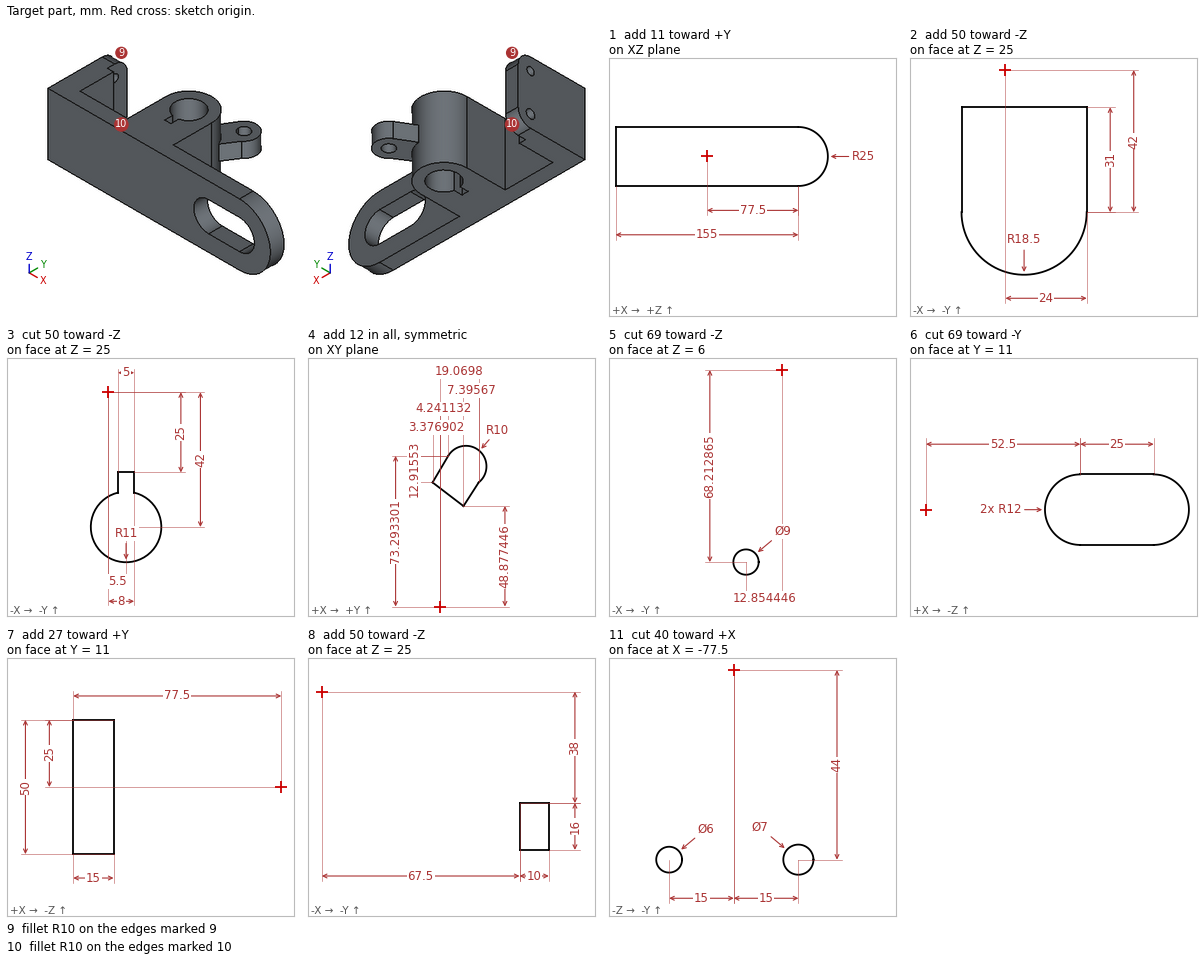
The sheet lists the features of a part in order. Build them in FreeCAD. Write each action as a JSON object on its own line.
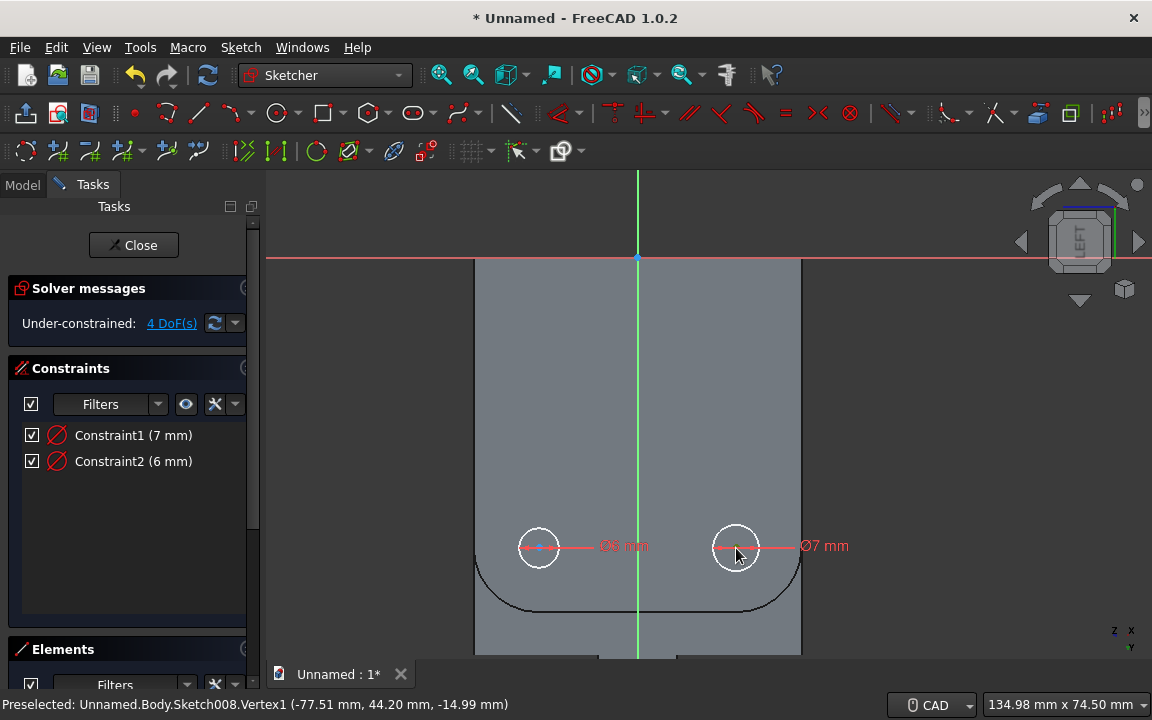
{"action": "left_click", "coordinate": [539, 548]}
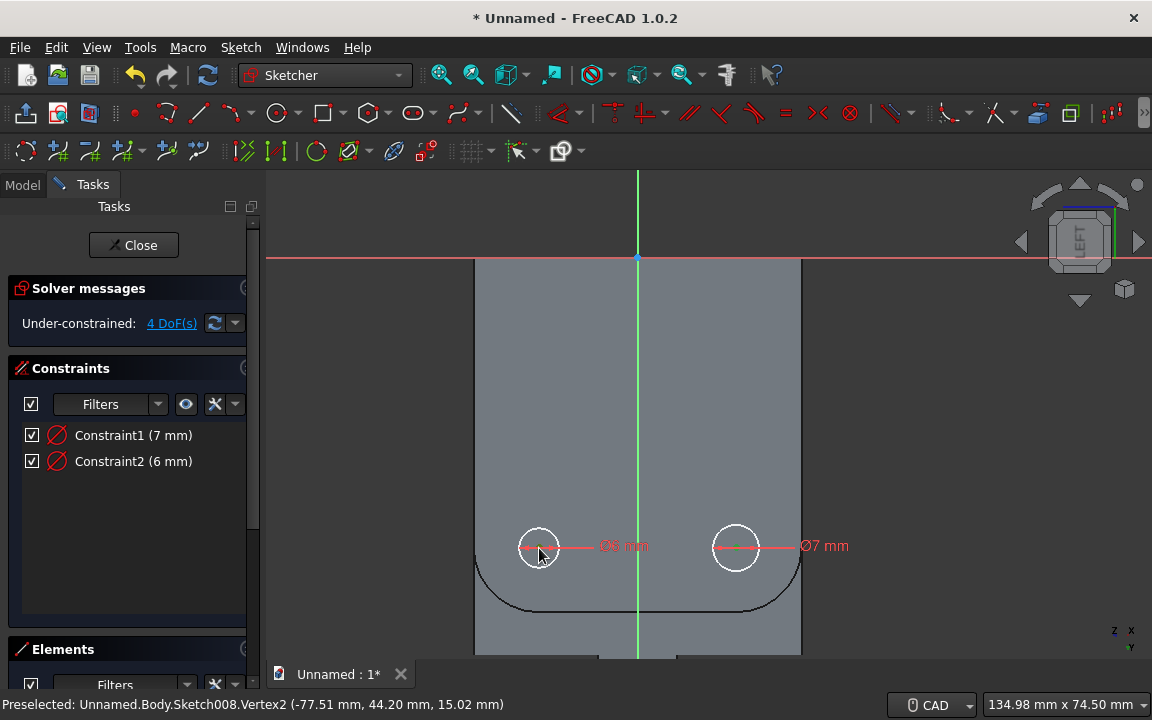
{"action": "left_click", "coordinate": [668, 114]}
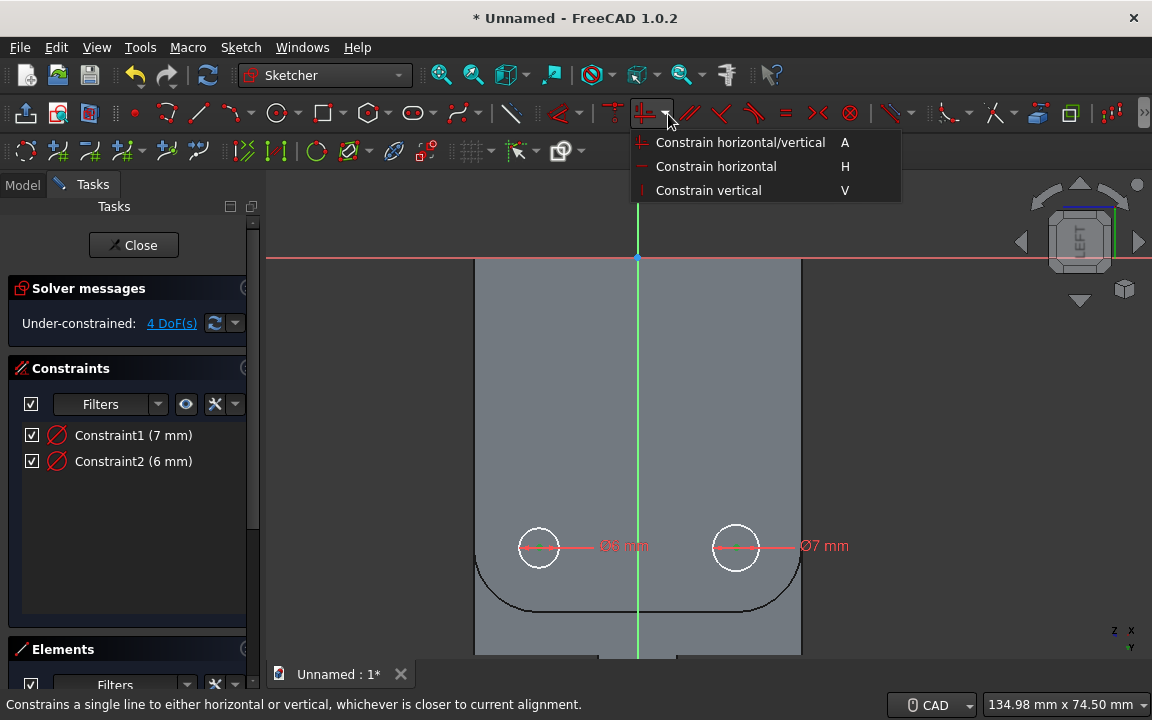
{"action": "left_click", "coordinate": [766, 166]}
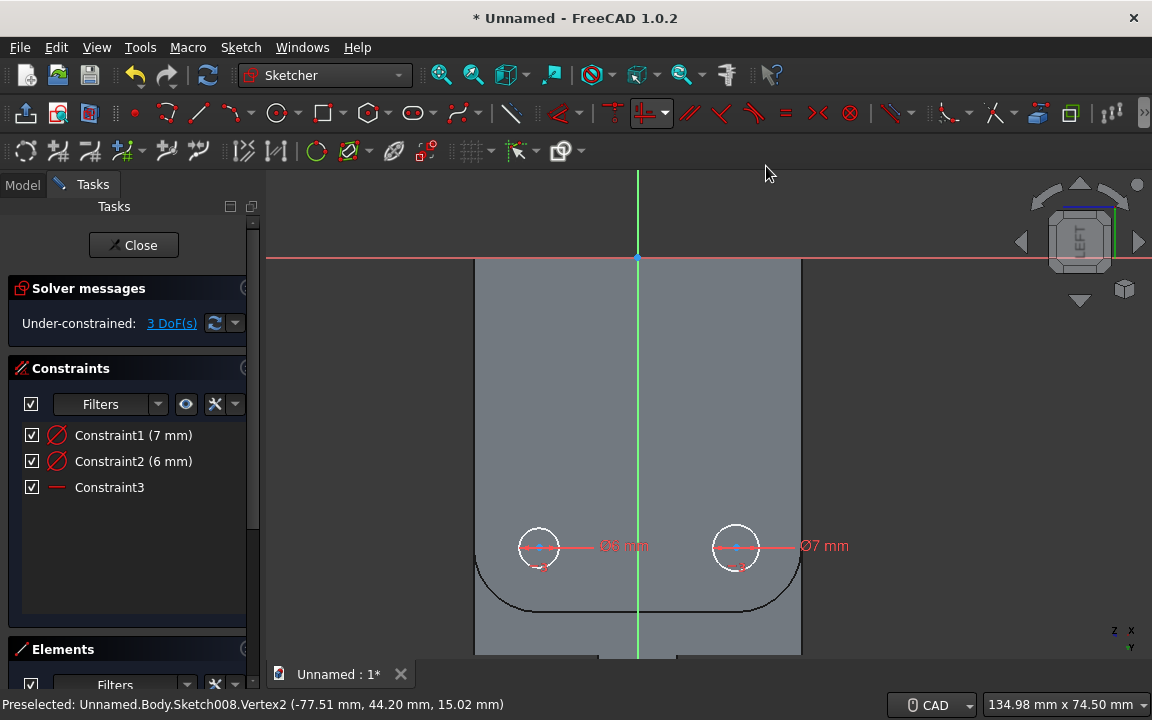
{"action": "left_click", "coordinate": [558, 114]}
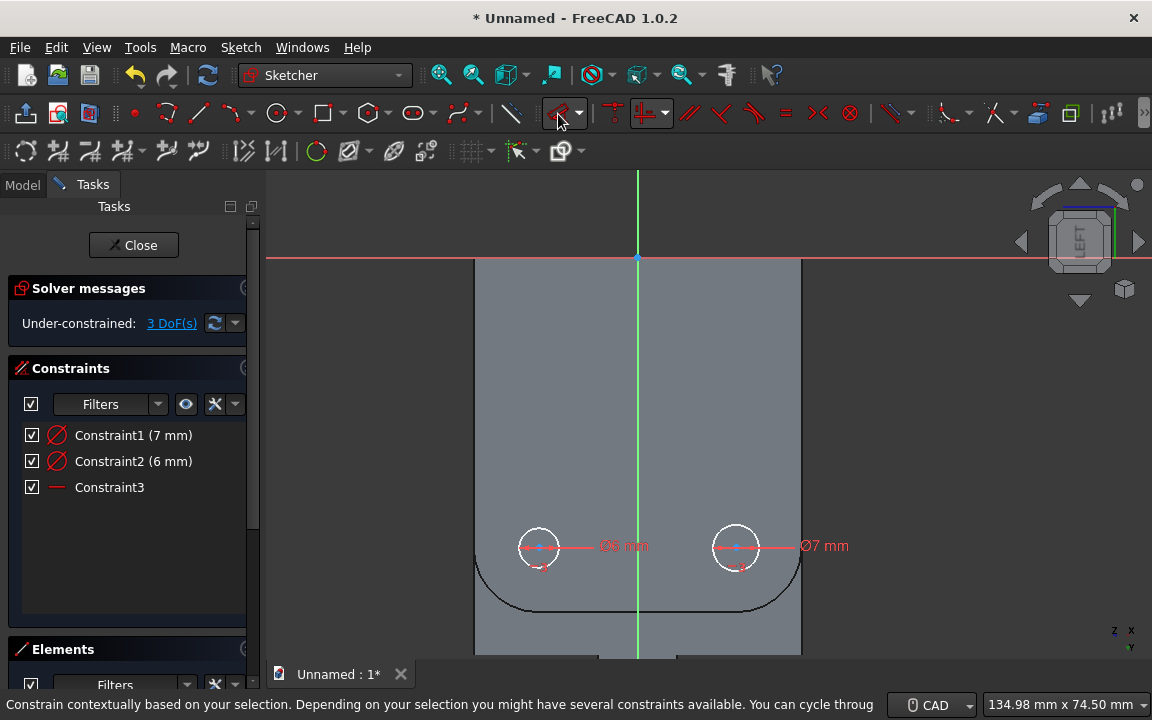
{"action": "left_click", "coordinate": [736, 548]}
{"action": "left_click", "coordinate": [687, 224]}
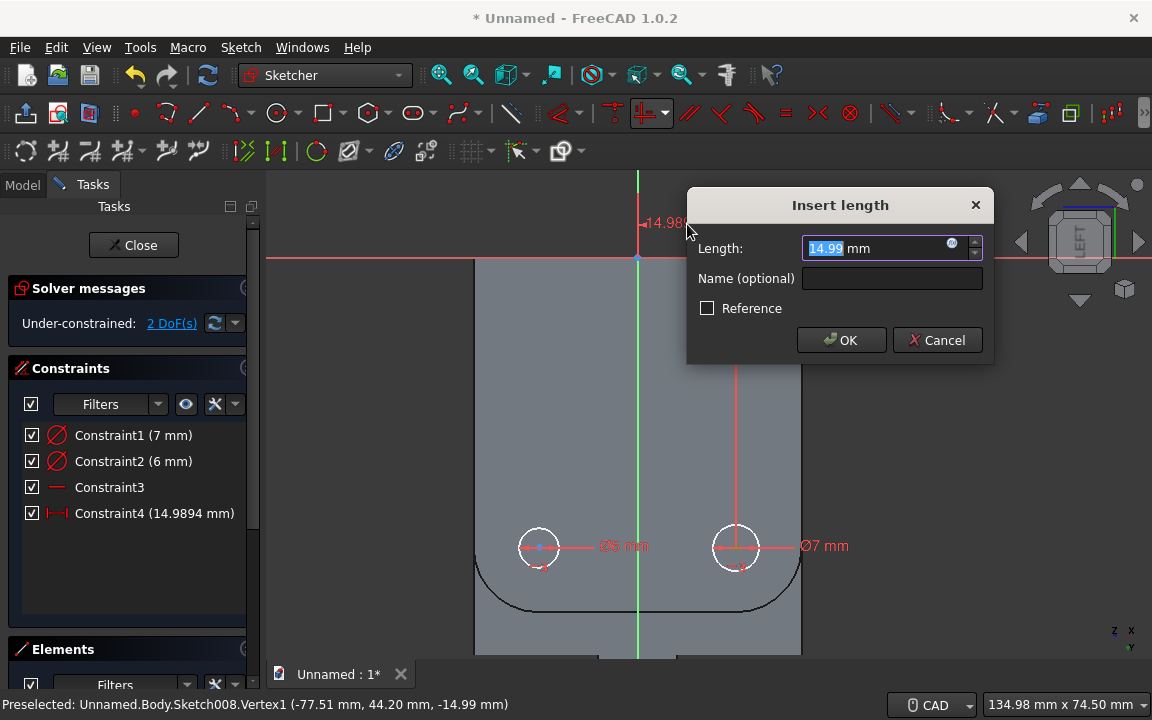
{"action": "type", "text": "15"}
{"action": "key", "text": "Return"}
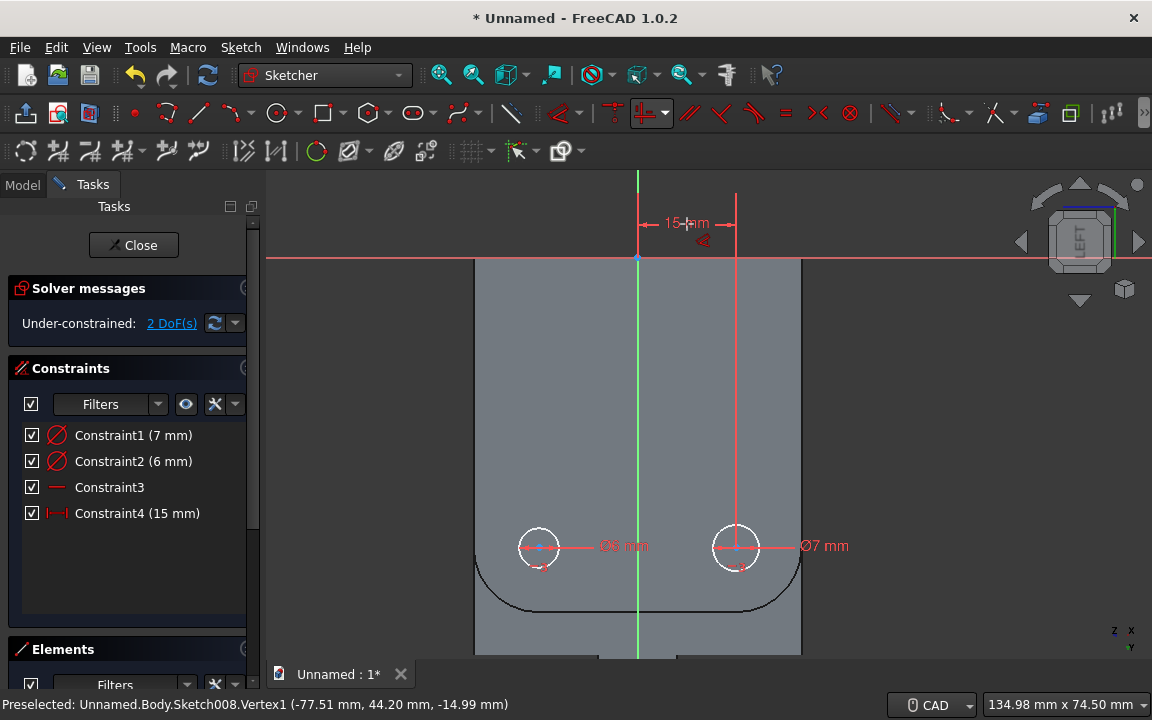
{"action": "left_click", "coordinate": [736, 548]}
{"action": "left_click", "coordinate": [770, 403]}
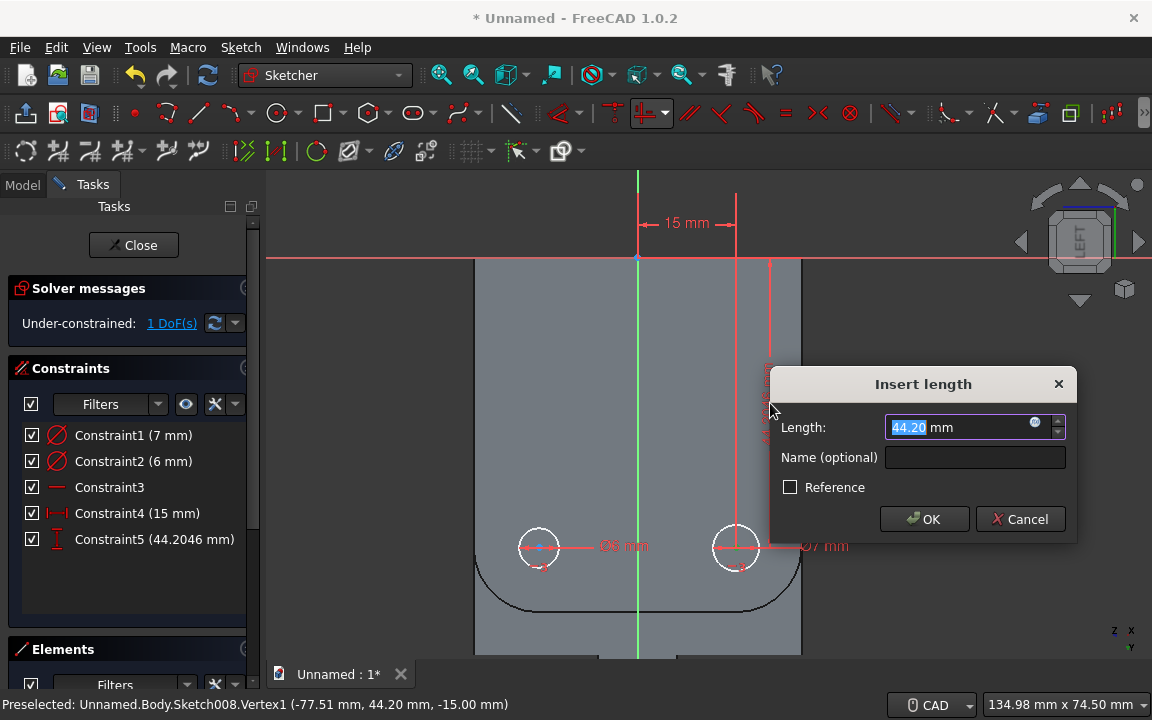
{"action": "type", "text": "44"}
{"action": "key", "text": "Return"}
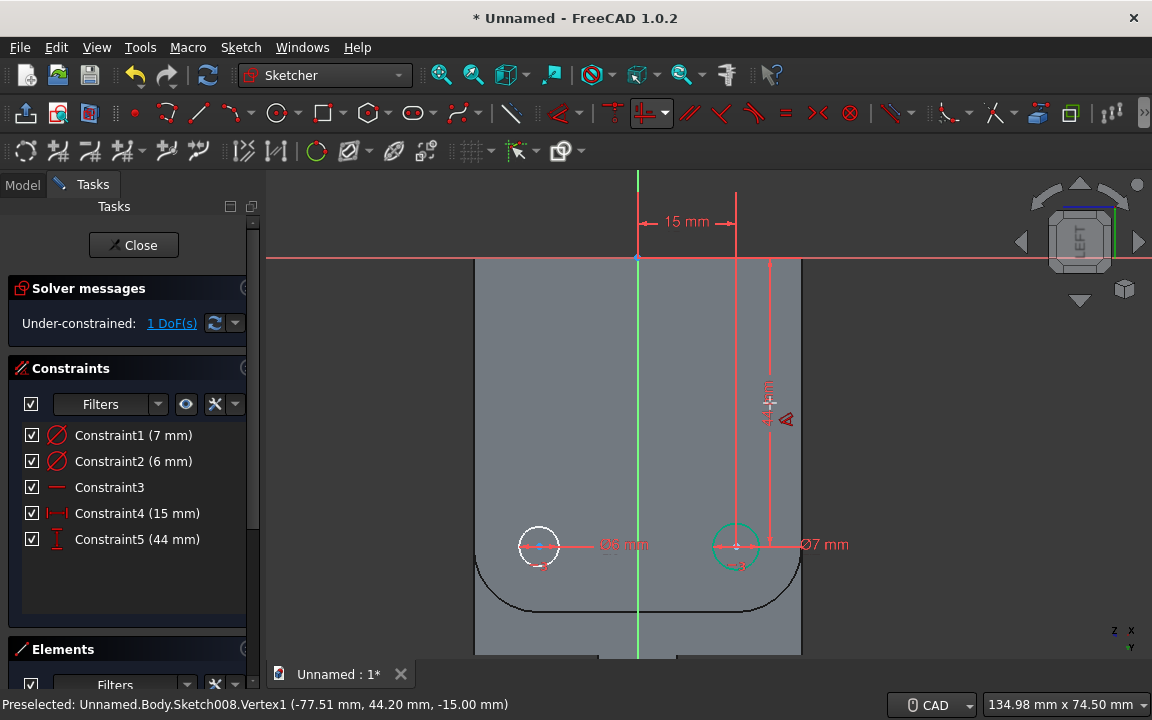
{"action": "left_click", "coordinate": [539, 547]}
{"action": "left_click", "coordinate": [588, 224]}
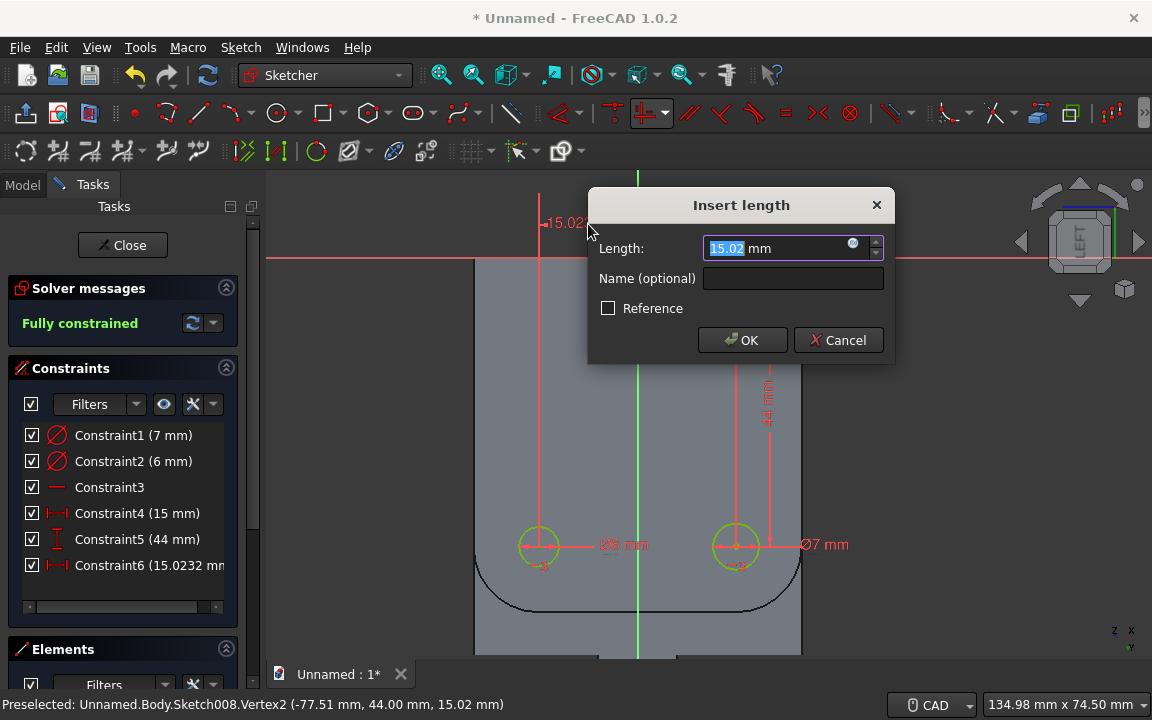
{"action": "type", "text": "15"}
{"action": "key", "text": "Return"}
{"action": "key", "text": "Escape"}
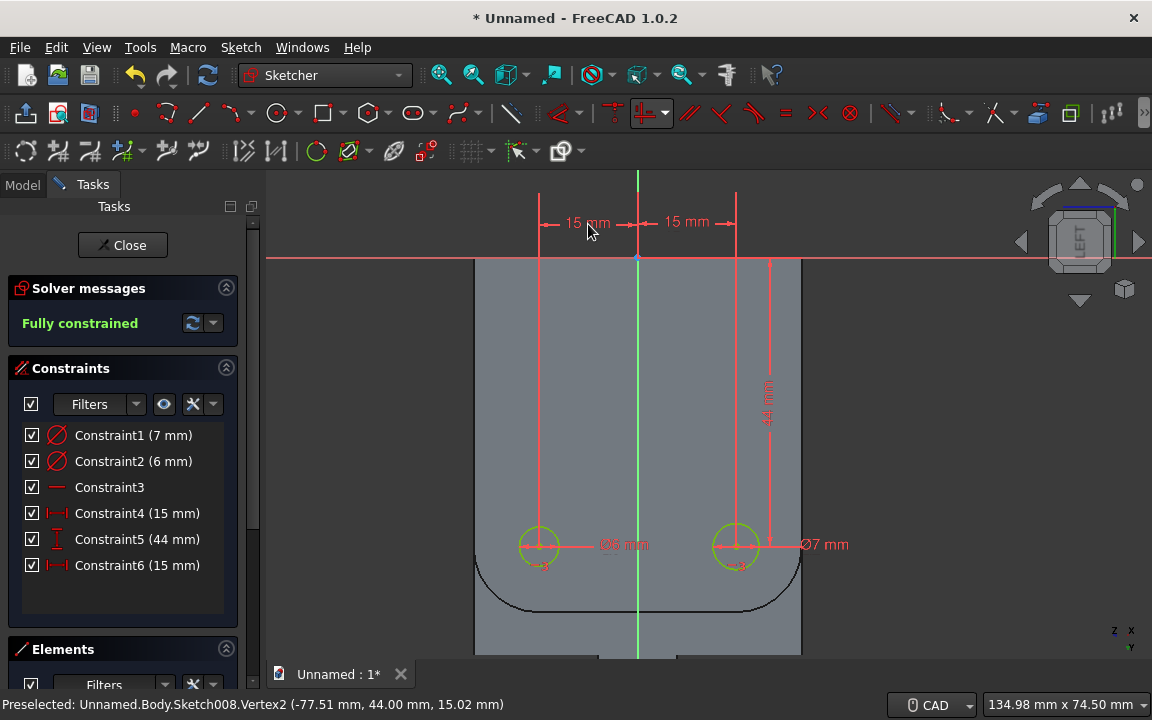
{"action": "left_click", "coordinate": [123, 245]}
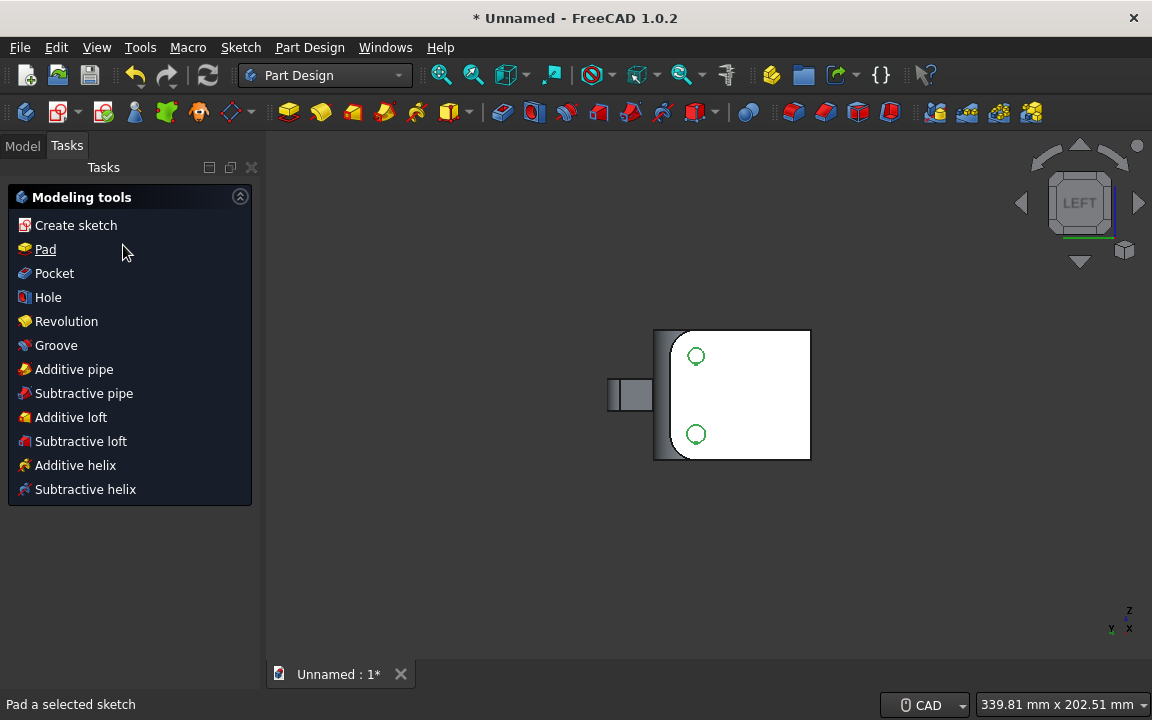
{"action": "left_click", "coordinate": [504, 112]}